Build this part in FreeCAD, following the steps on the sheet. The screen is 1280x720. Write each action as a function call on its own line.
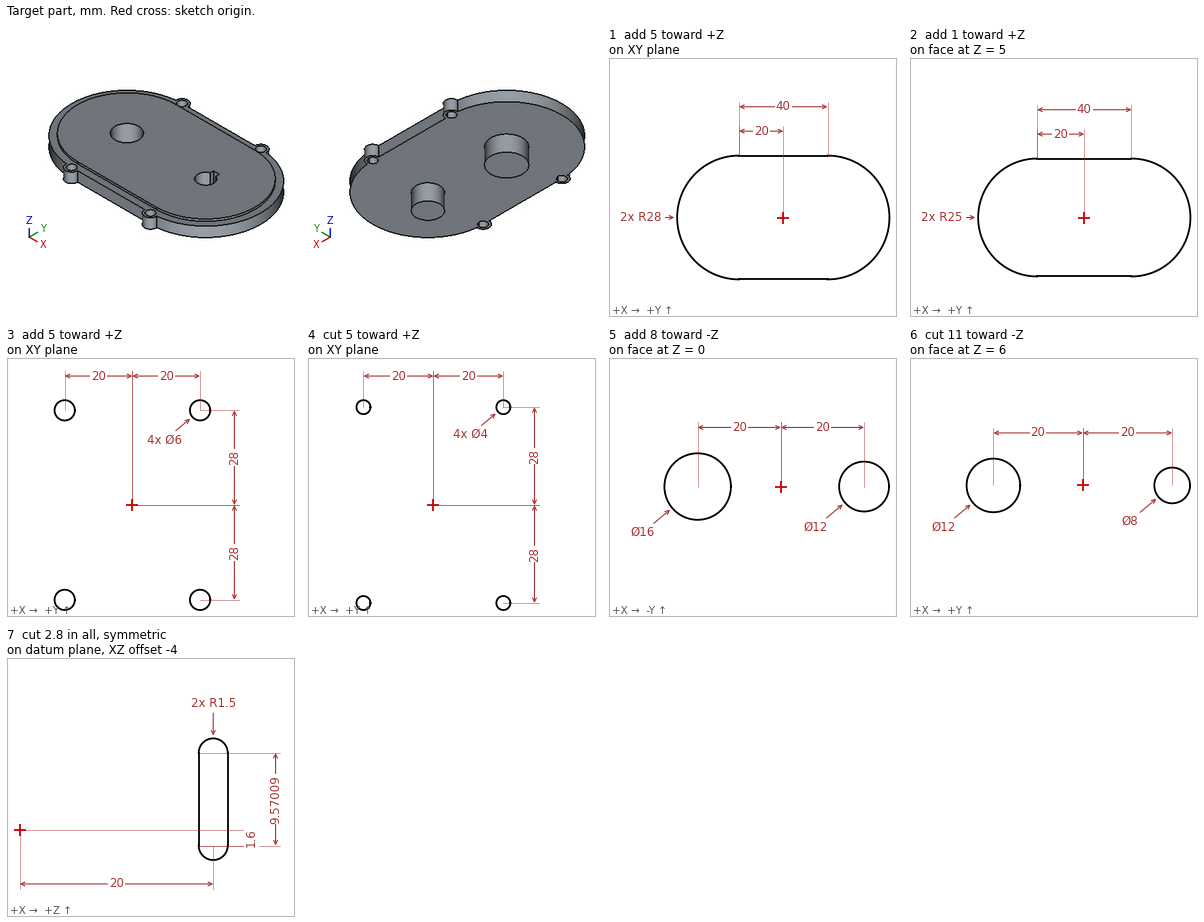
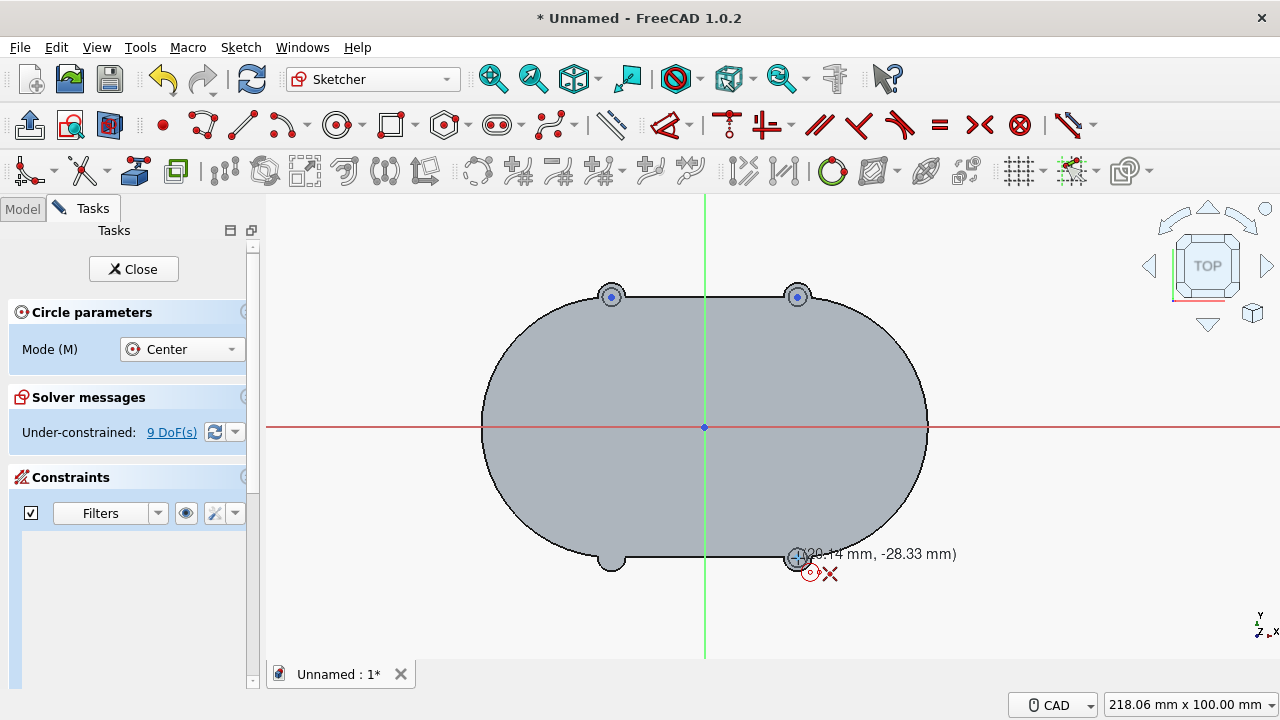
scroll(612, 557, up, 5)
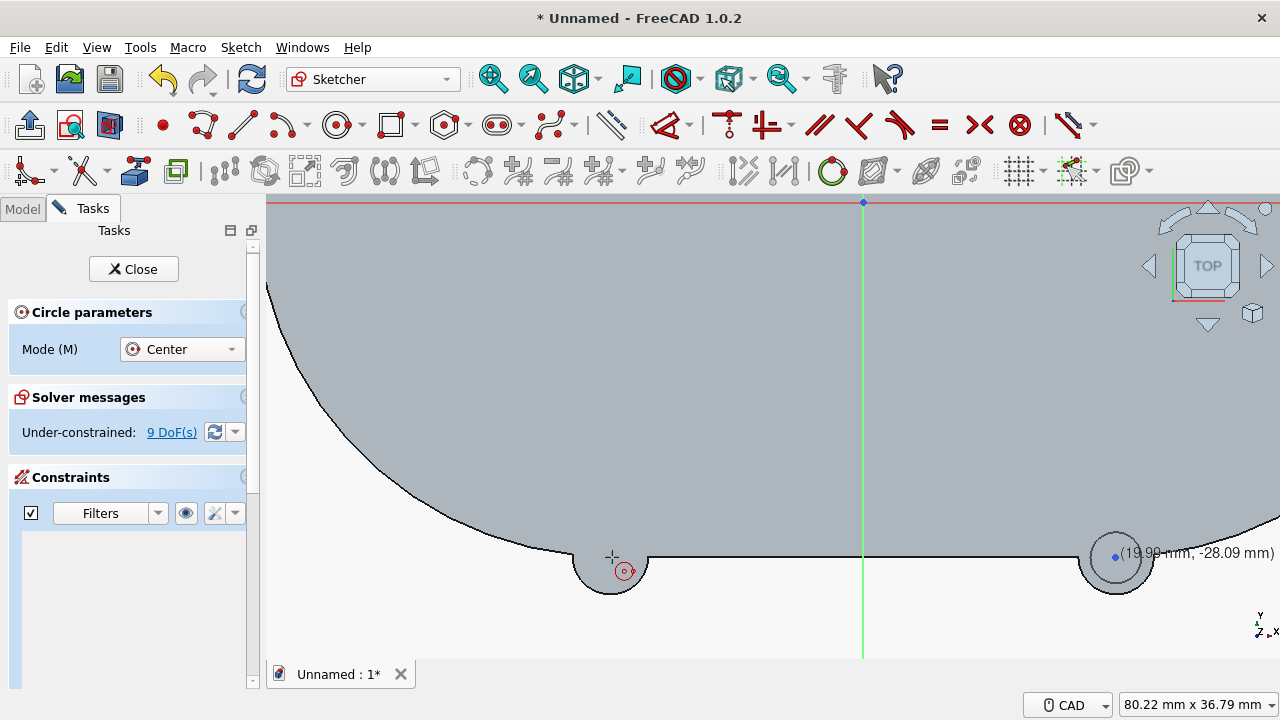
click(610, 557)
click(628, 539)
key(Escape)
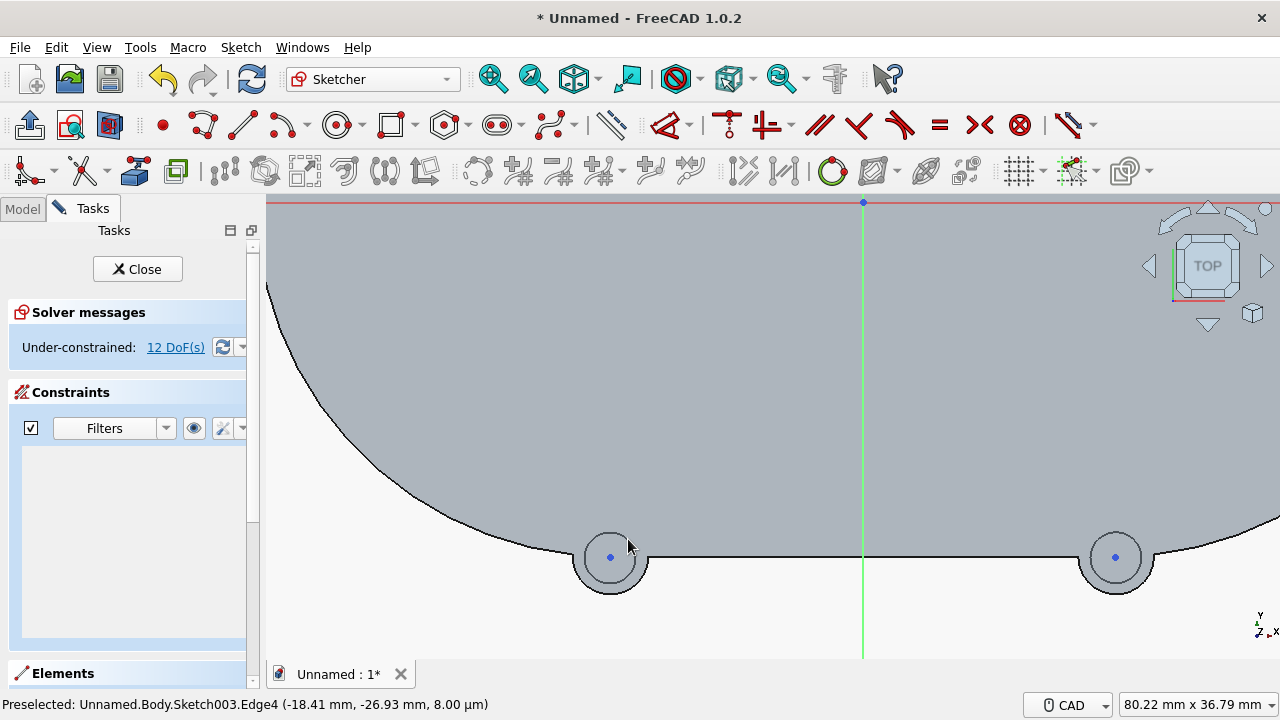
scroll(612, 557, down, 5)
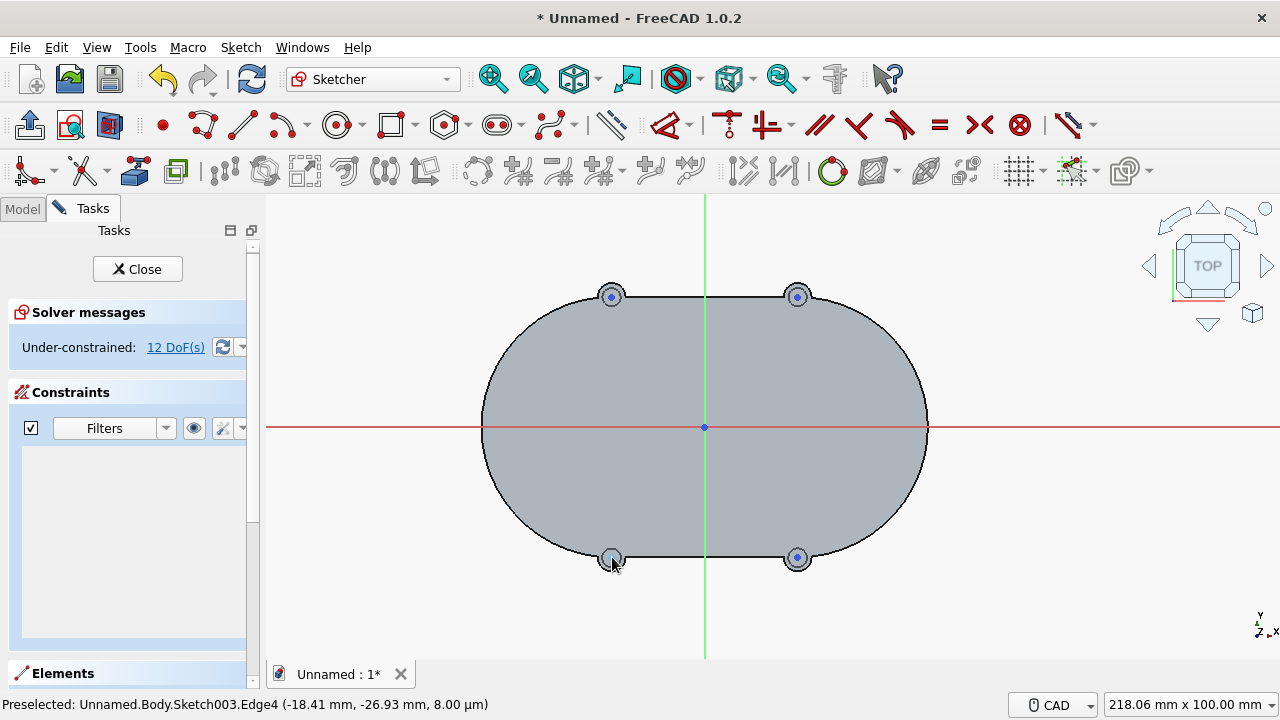
scroll(804, 291, up, 3)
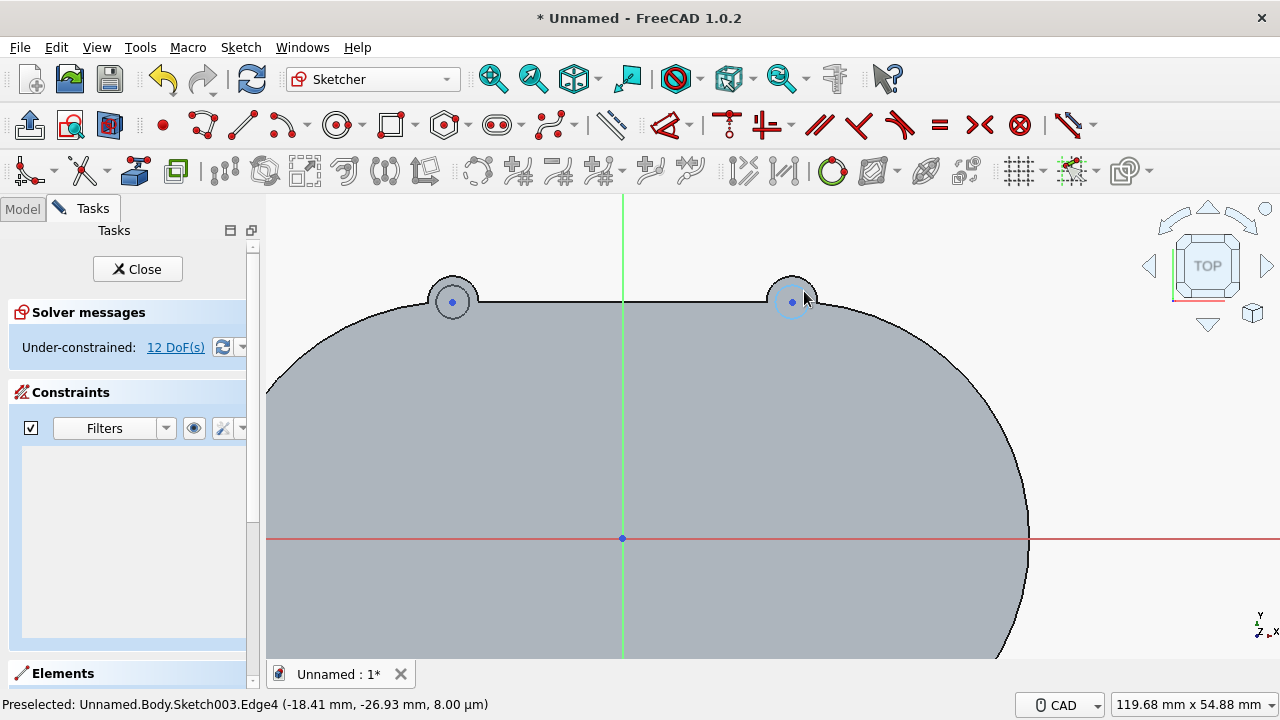
click(804, 290)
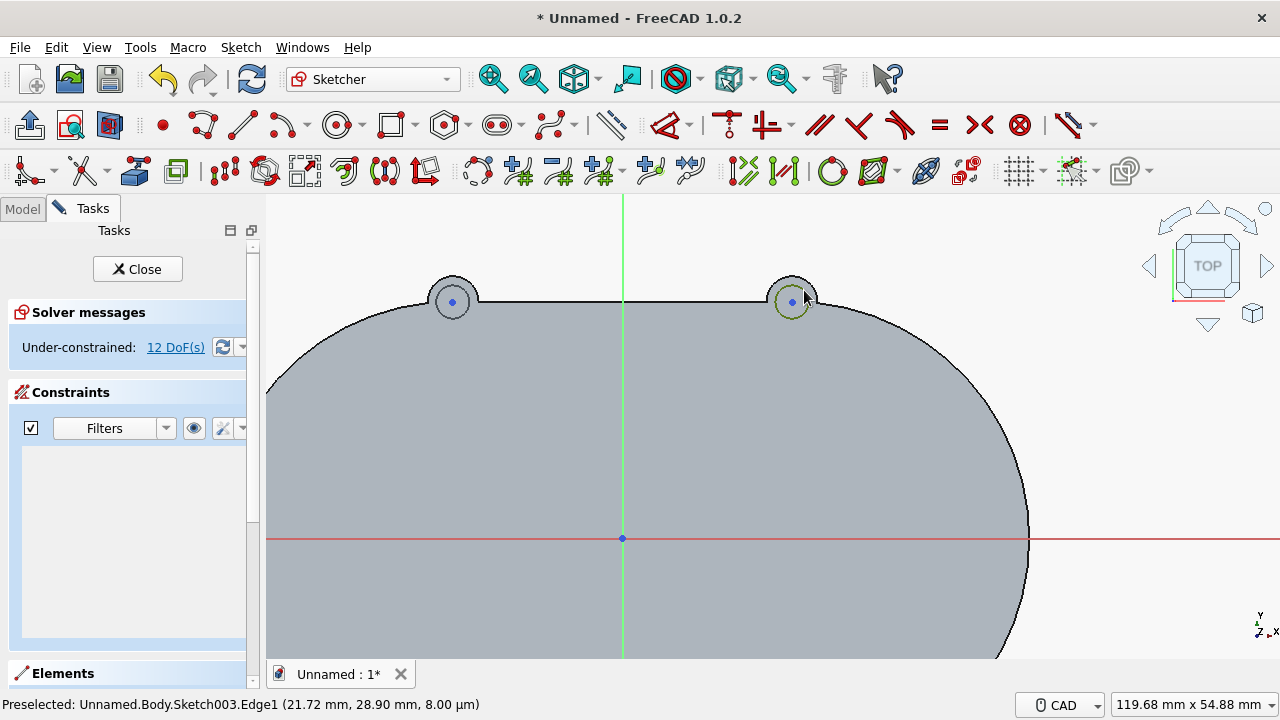
click(465, 290)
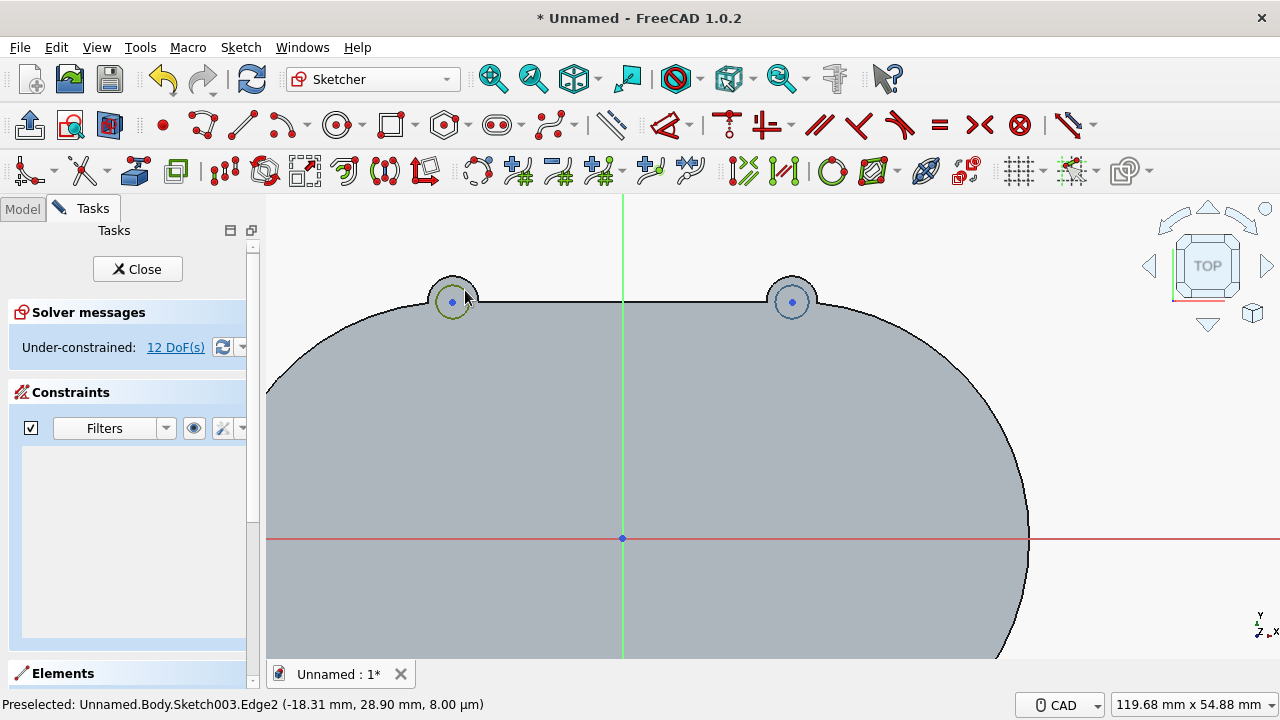
scroll(804, 290, down, 3)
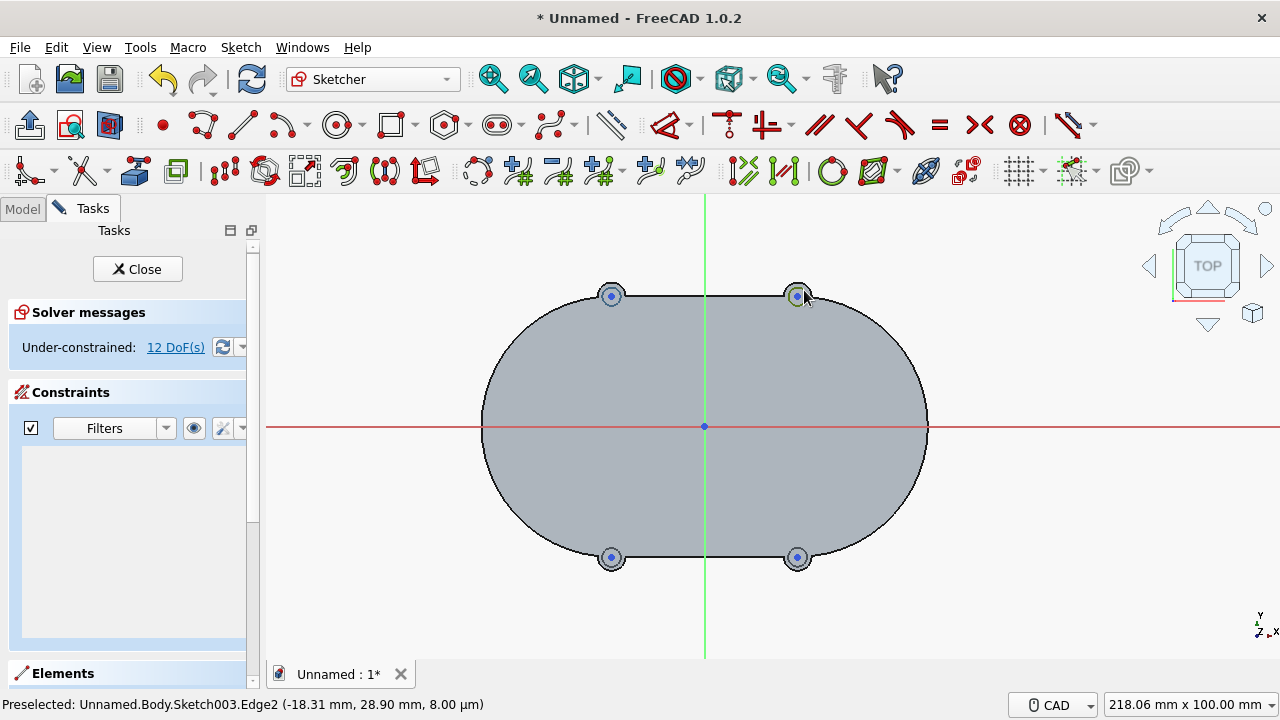
scroll(804, 551, up, 2)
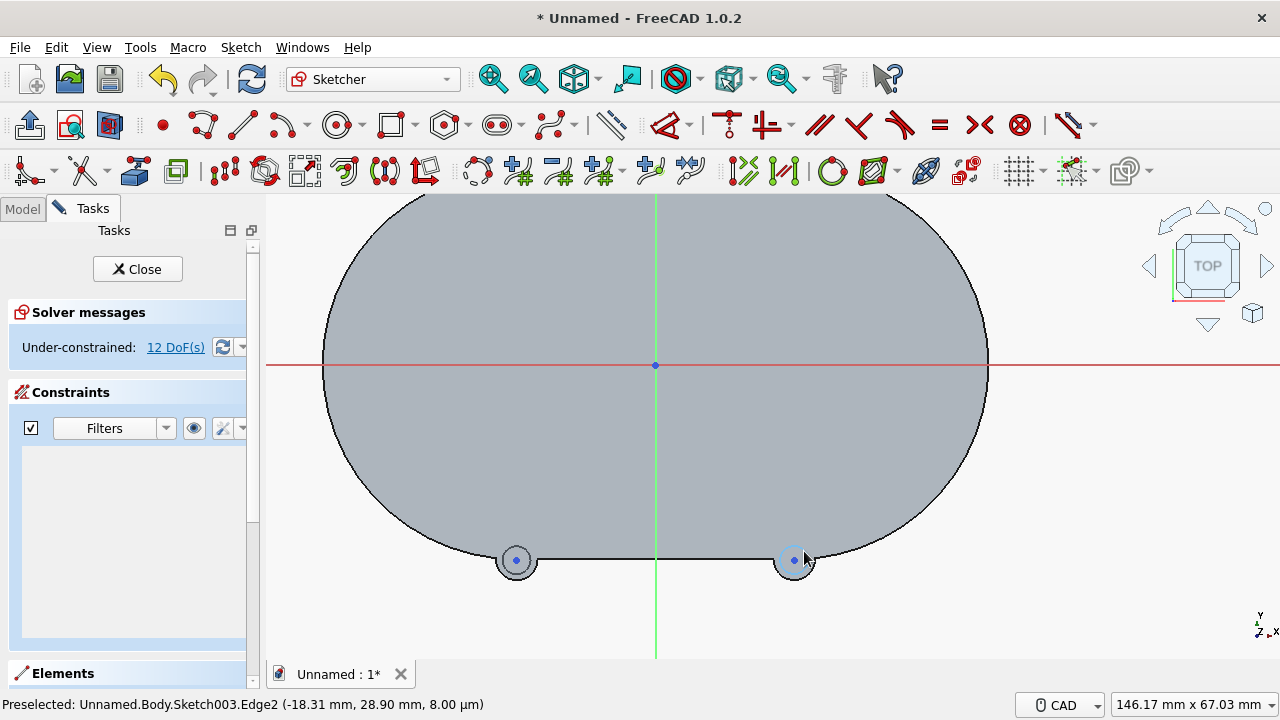
click(804, 550)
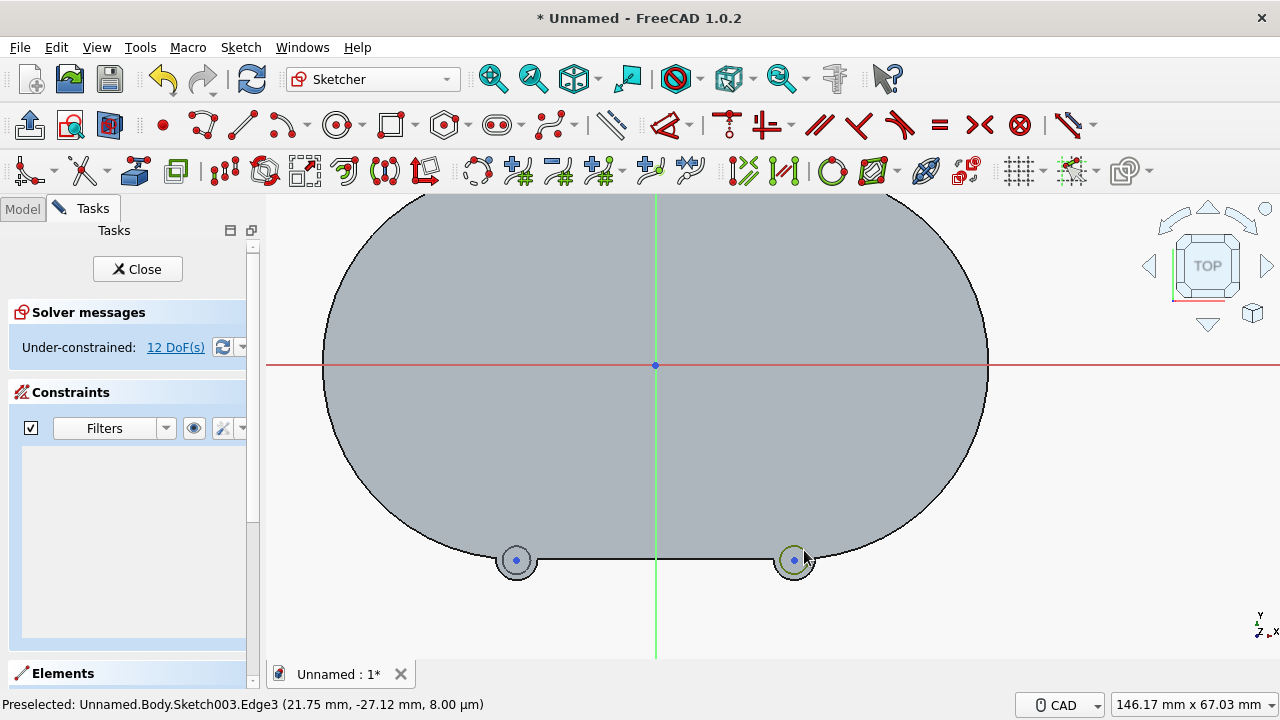
click(526, 550)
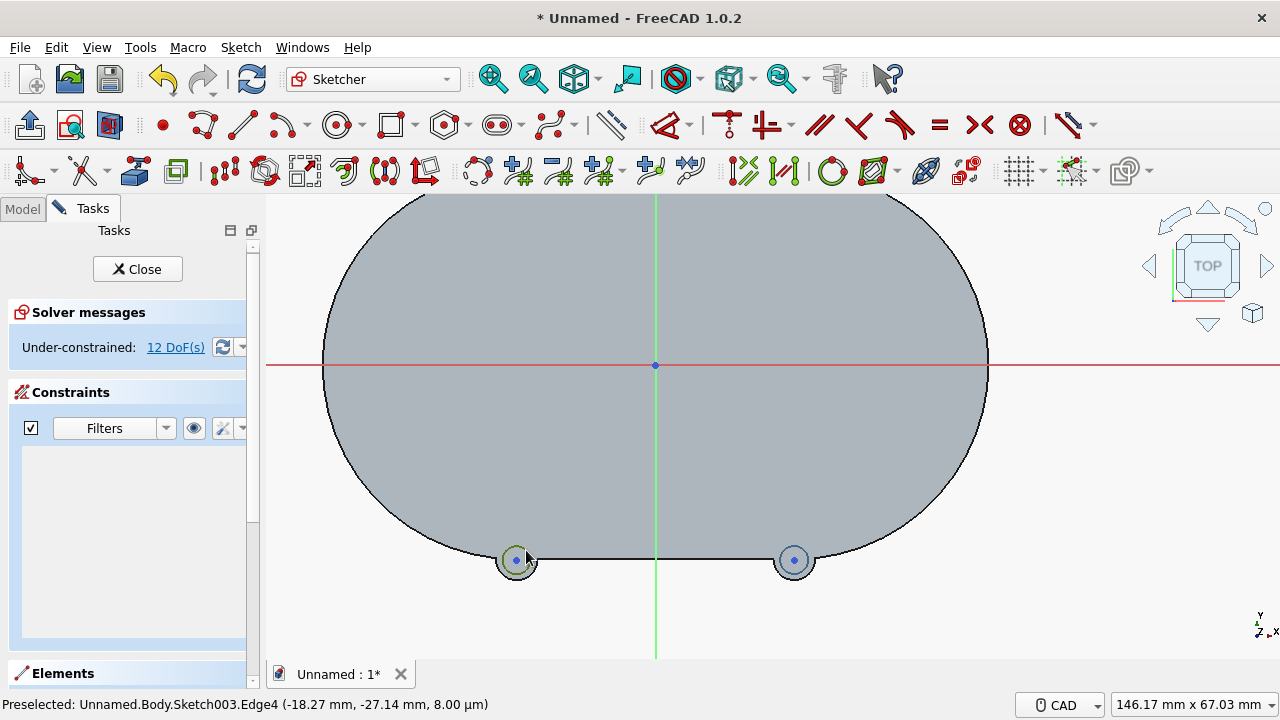
key(e)